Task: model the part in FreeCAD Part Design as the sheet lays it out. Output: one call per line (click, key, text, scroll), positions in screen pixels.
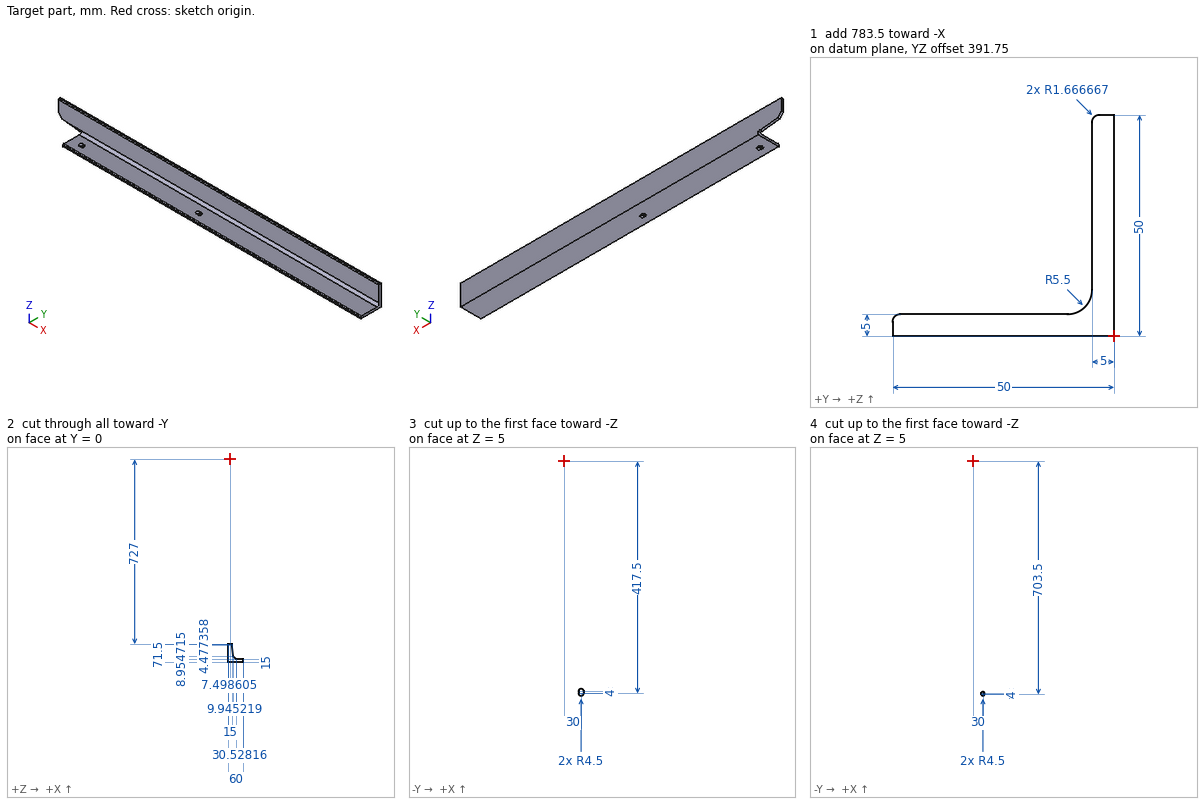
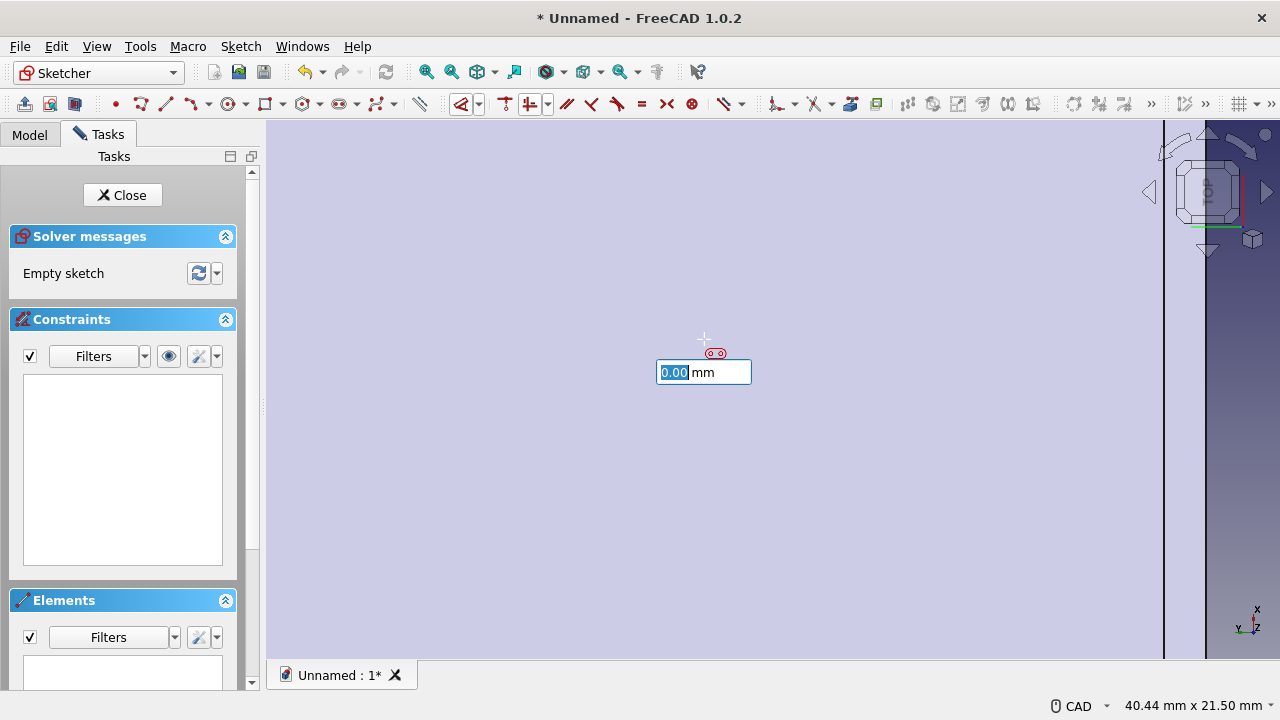
click(592, 389)
key(Escape)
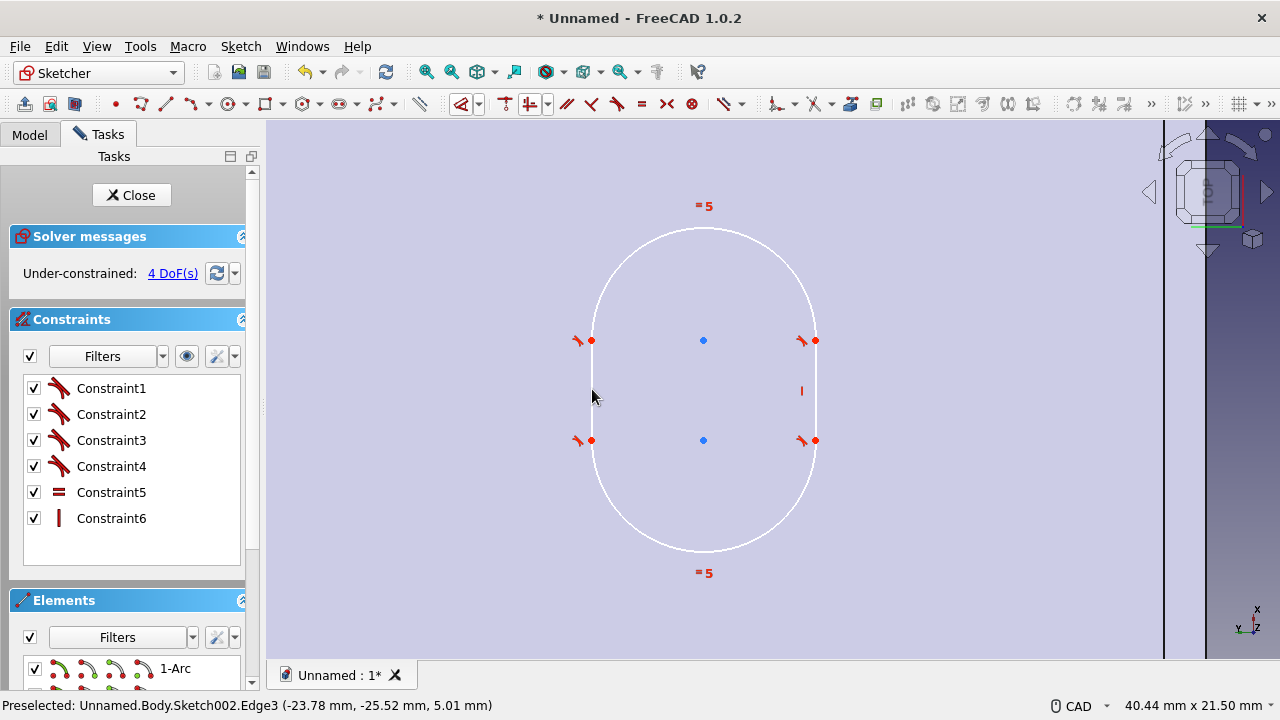
click(638, 531)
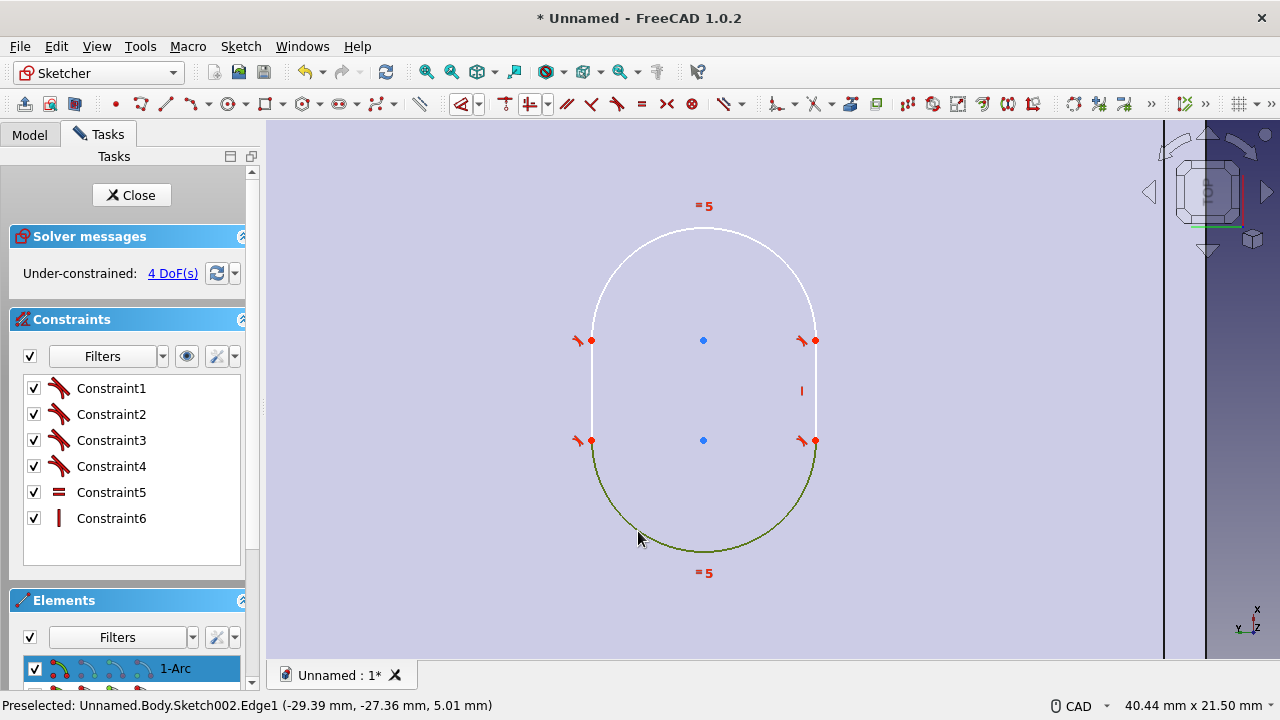
key(k)
key(r)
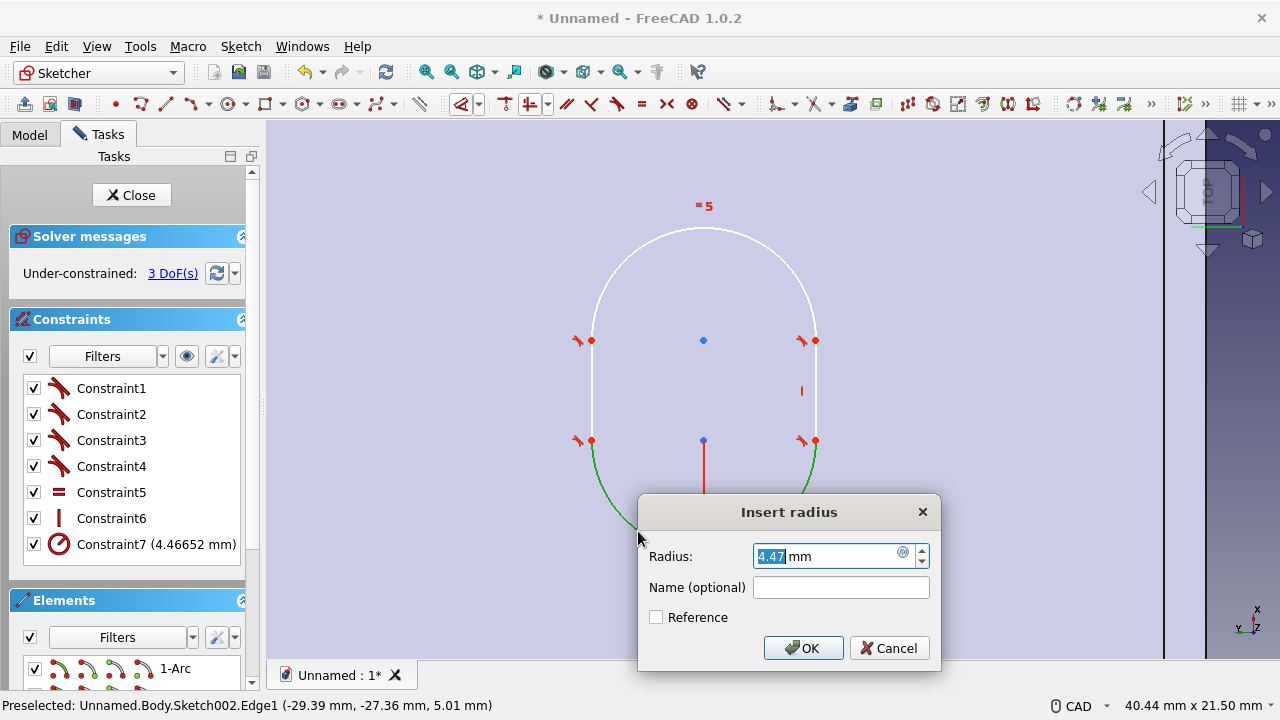
text(4.5)
key(Return)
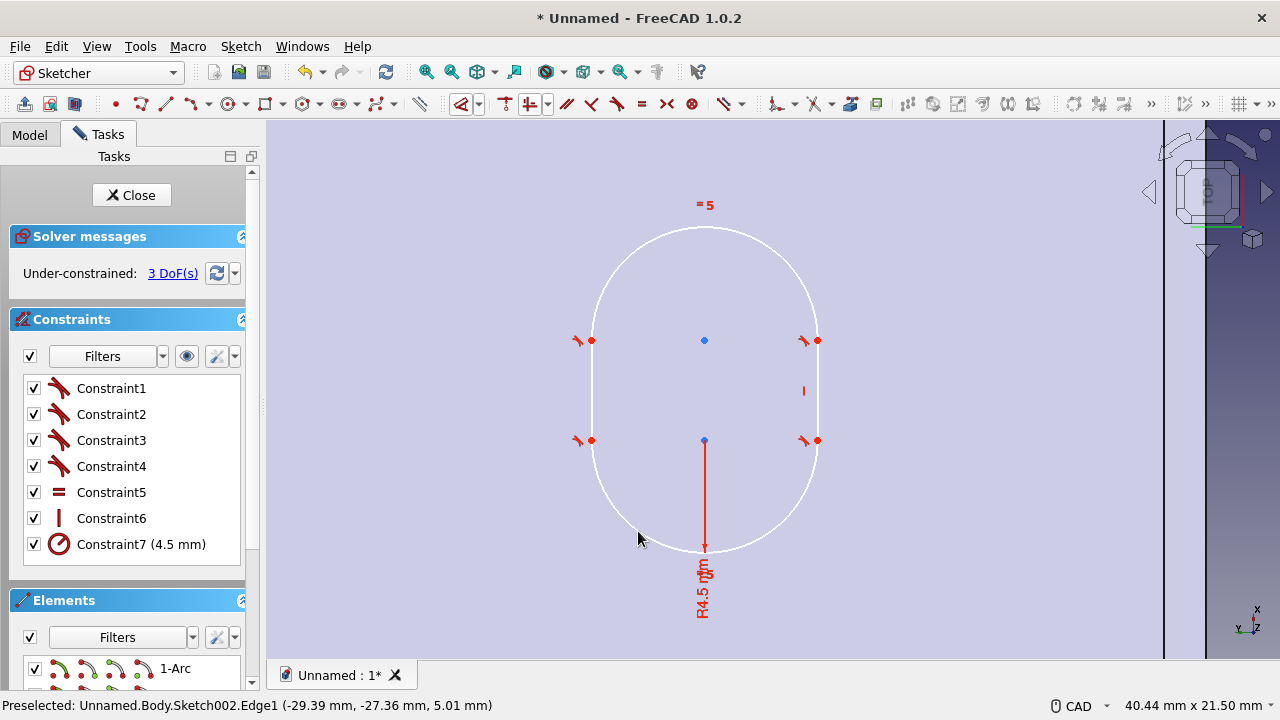
click(592, 410)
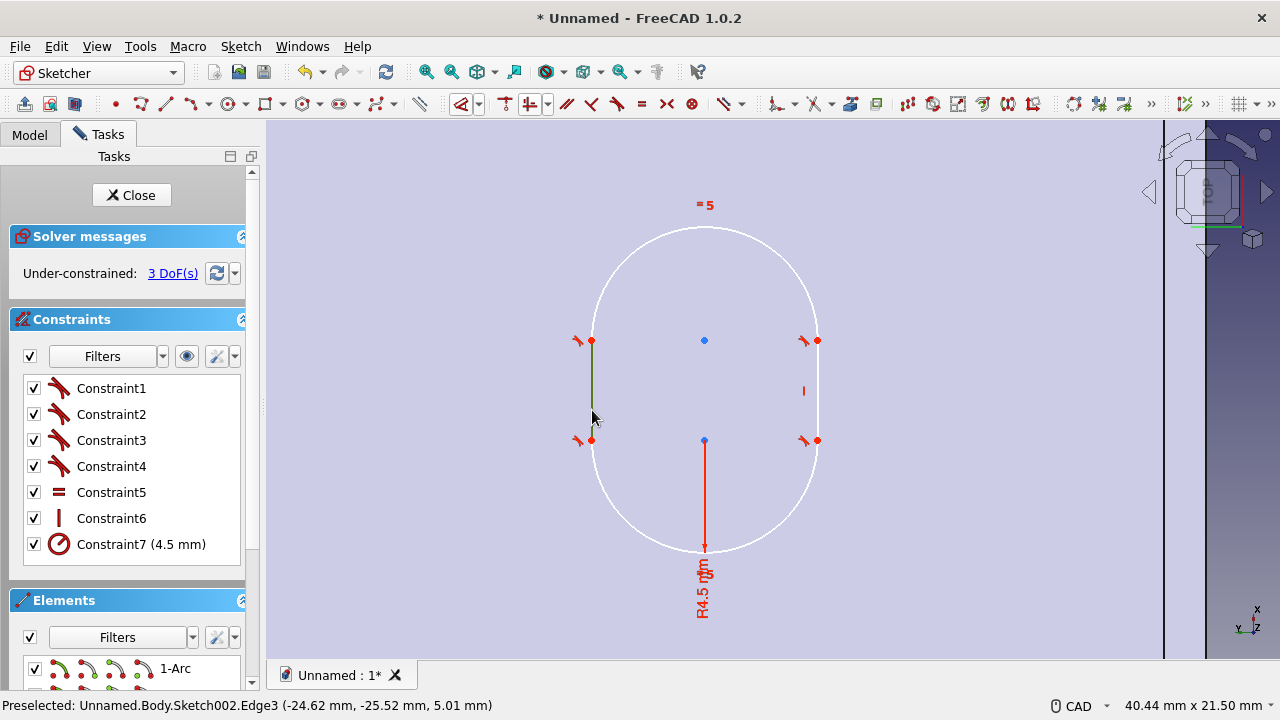
click(478, 104)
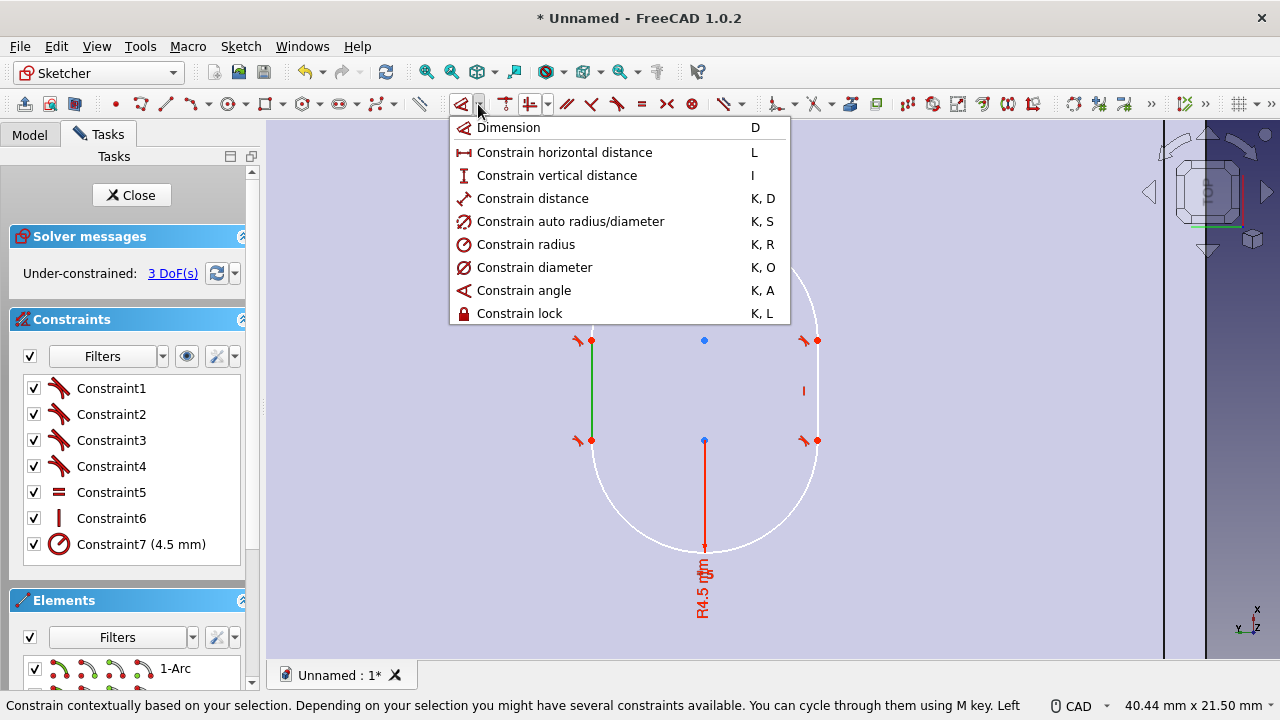
click(620, 176)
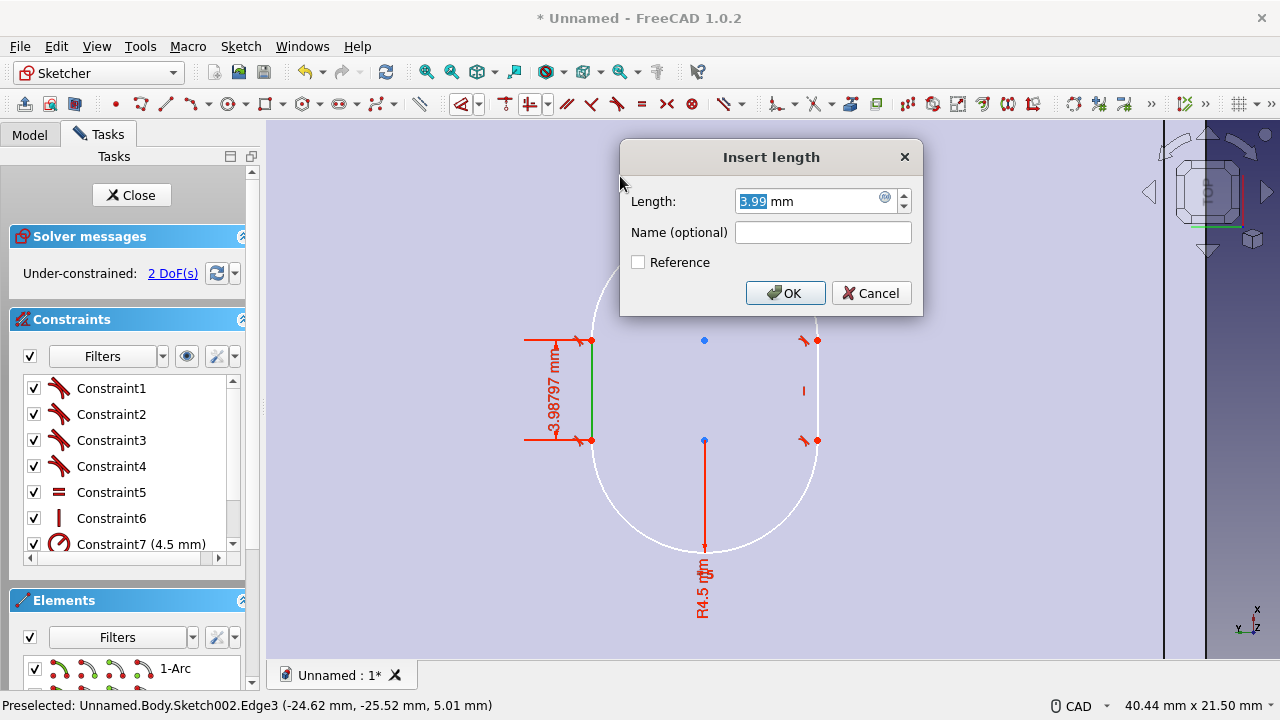
text(4)
key(Return)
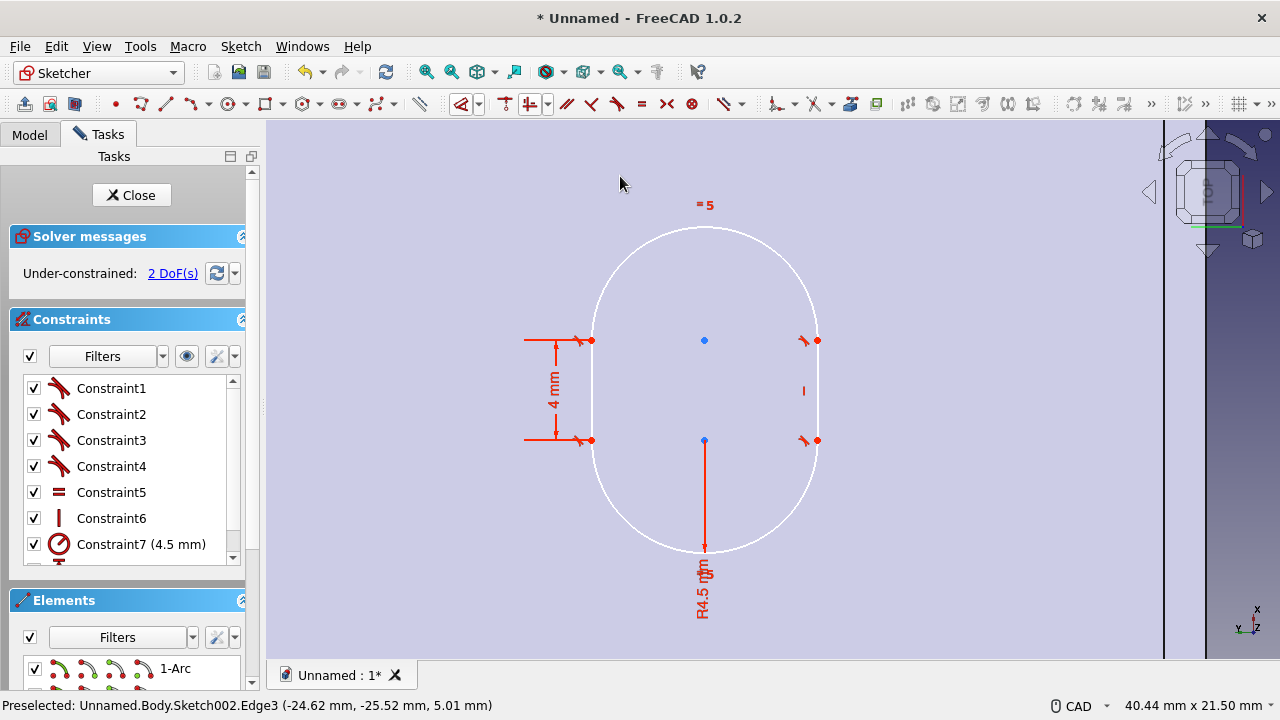
click(705, 440)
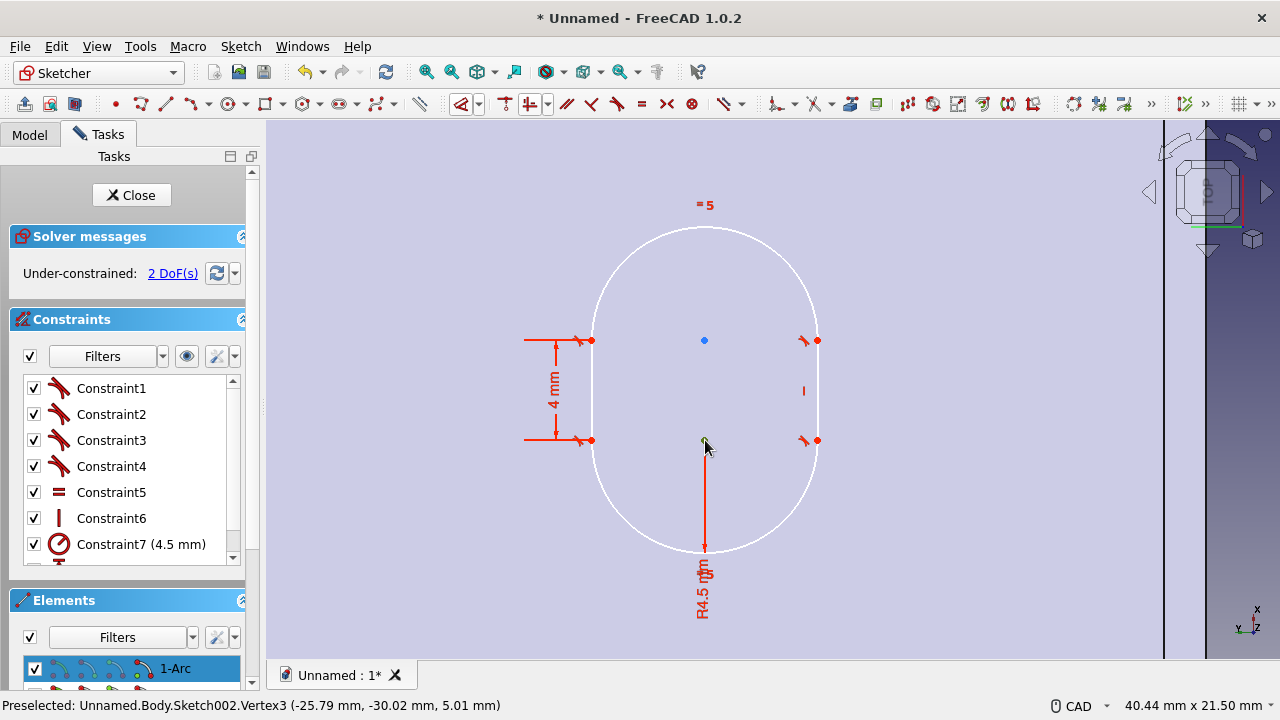
key(l)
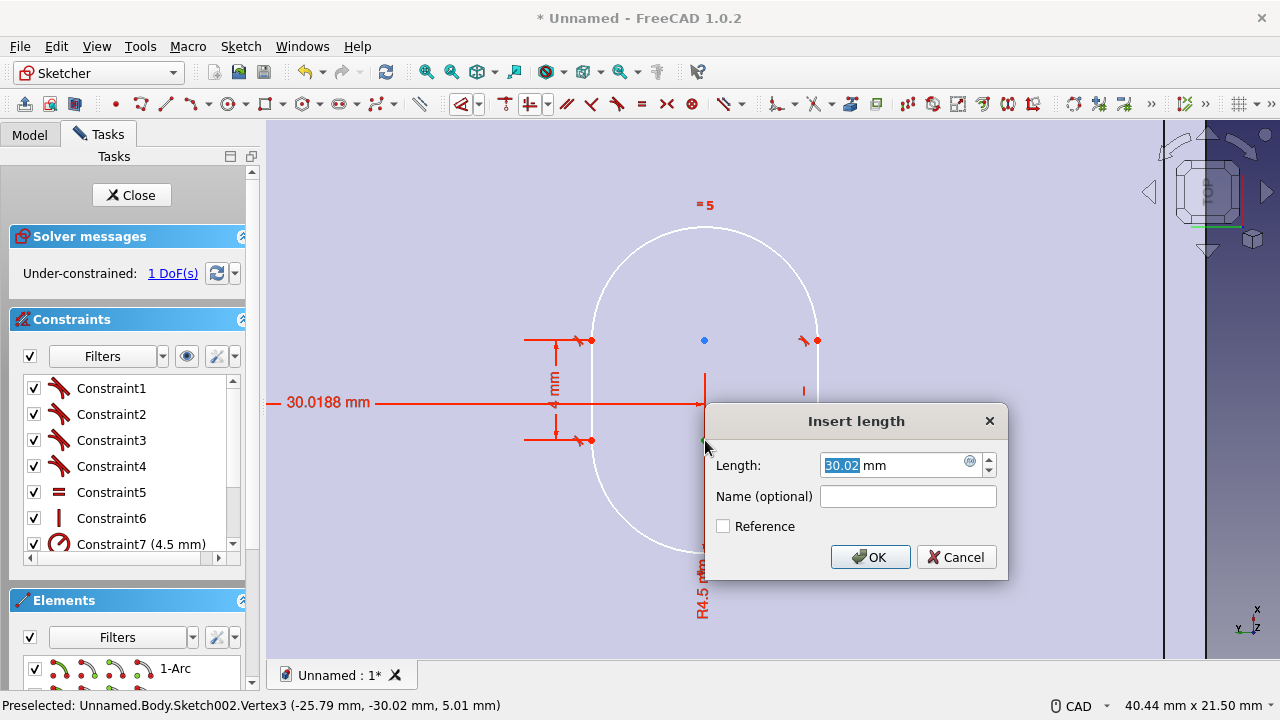
text(30)
key(Return)